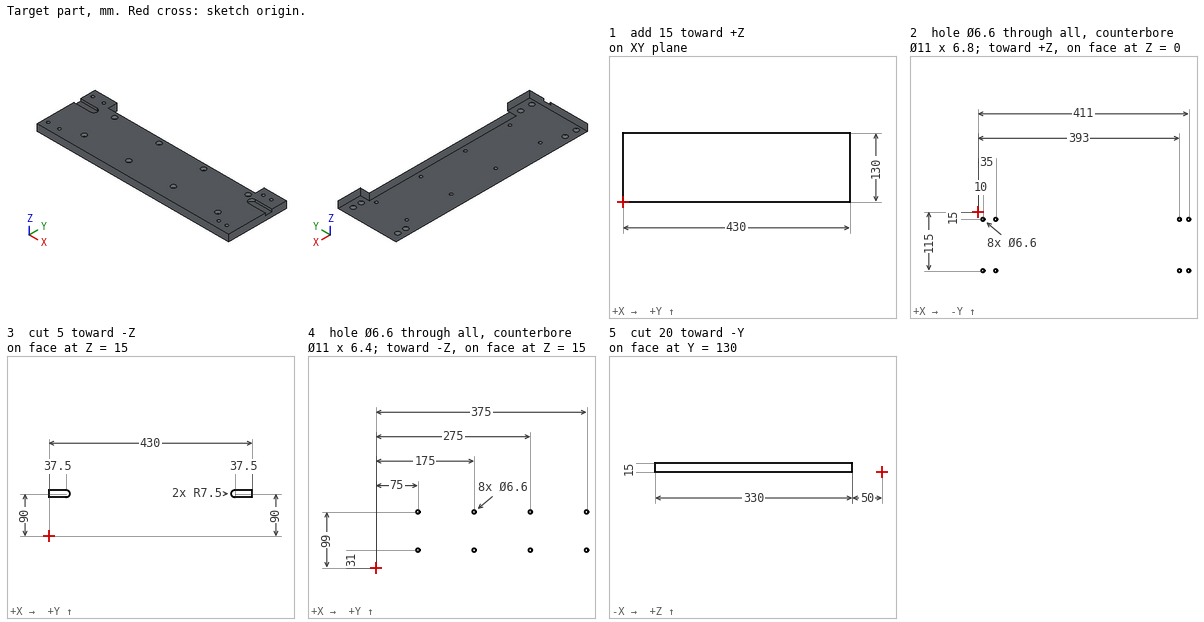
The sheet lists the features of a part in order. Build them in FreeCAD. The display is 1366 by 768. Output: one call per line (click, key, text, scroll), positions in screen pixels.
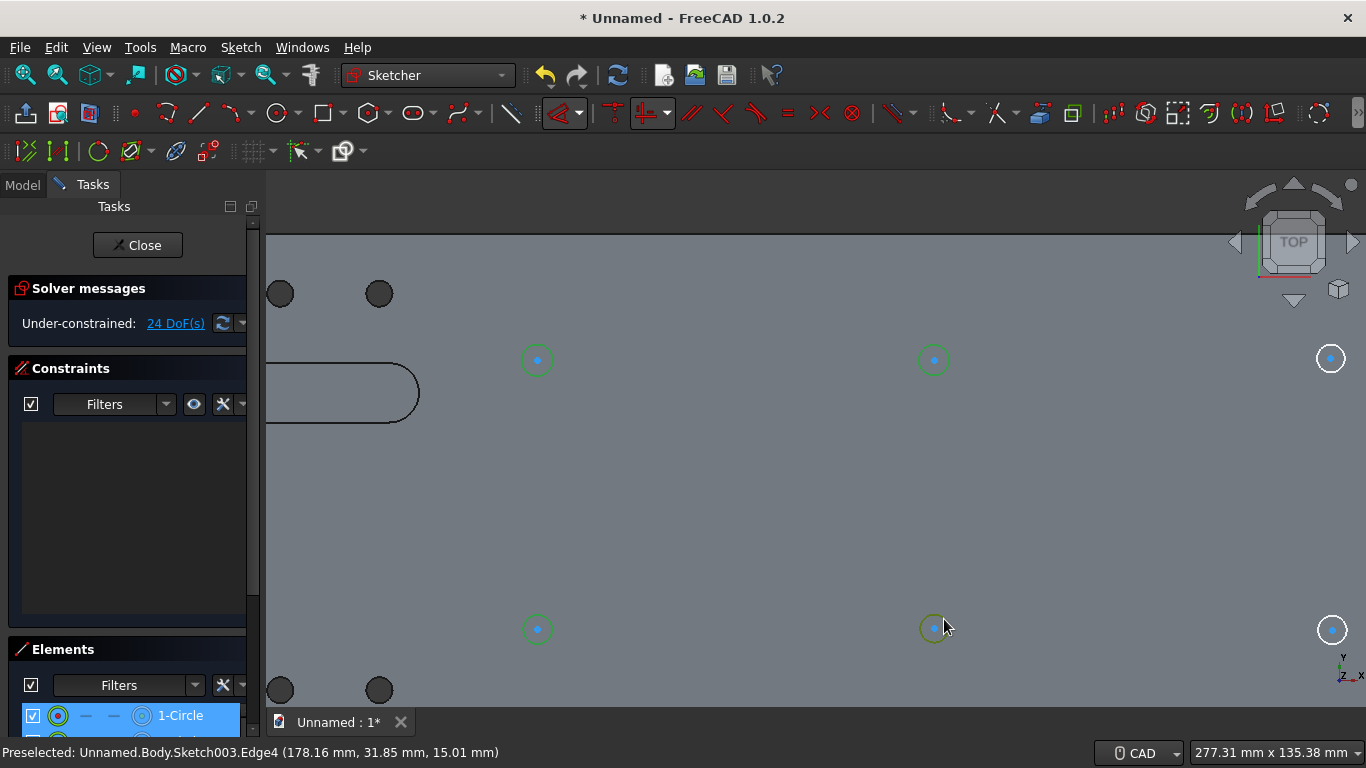
scroll(549, 350, down, 4)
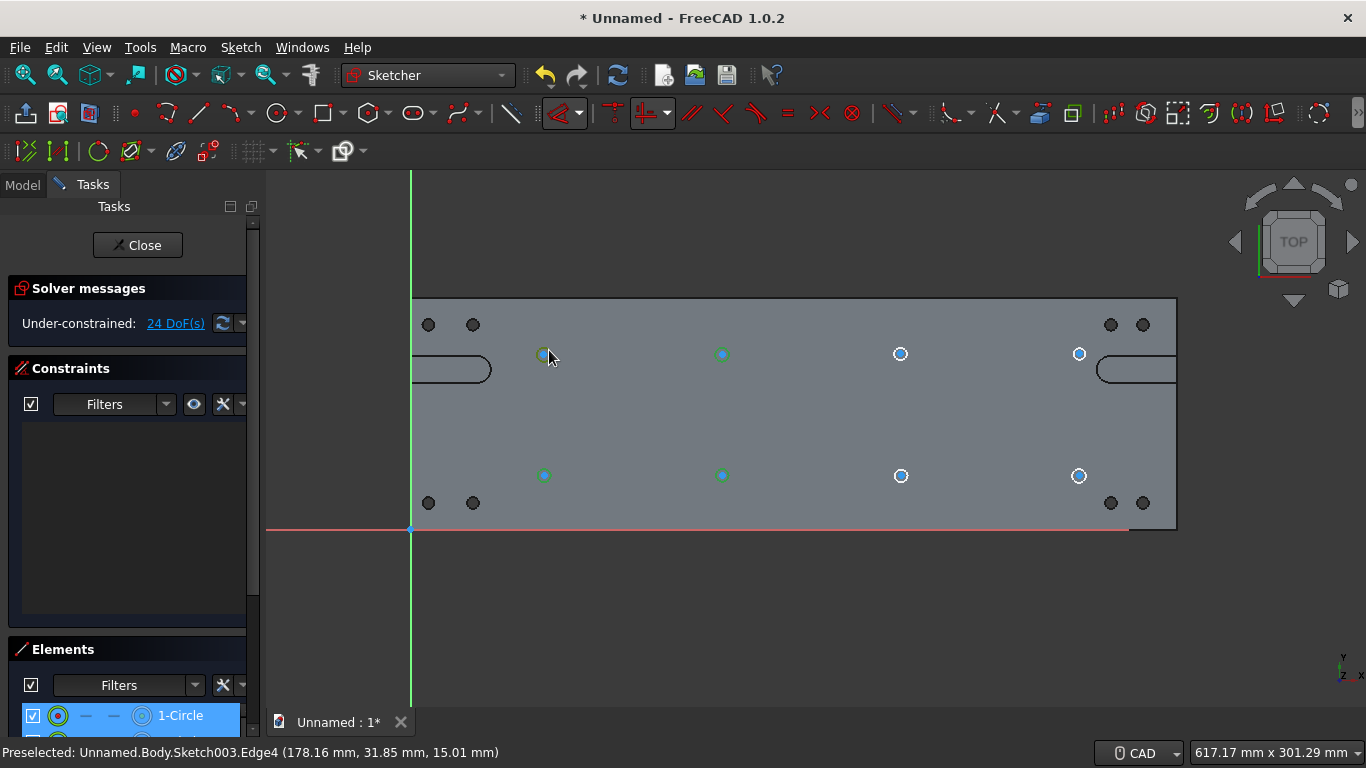
scroll(905, 350, up, 4)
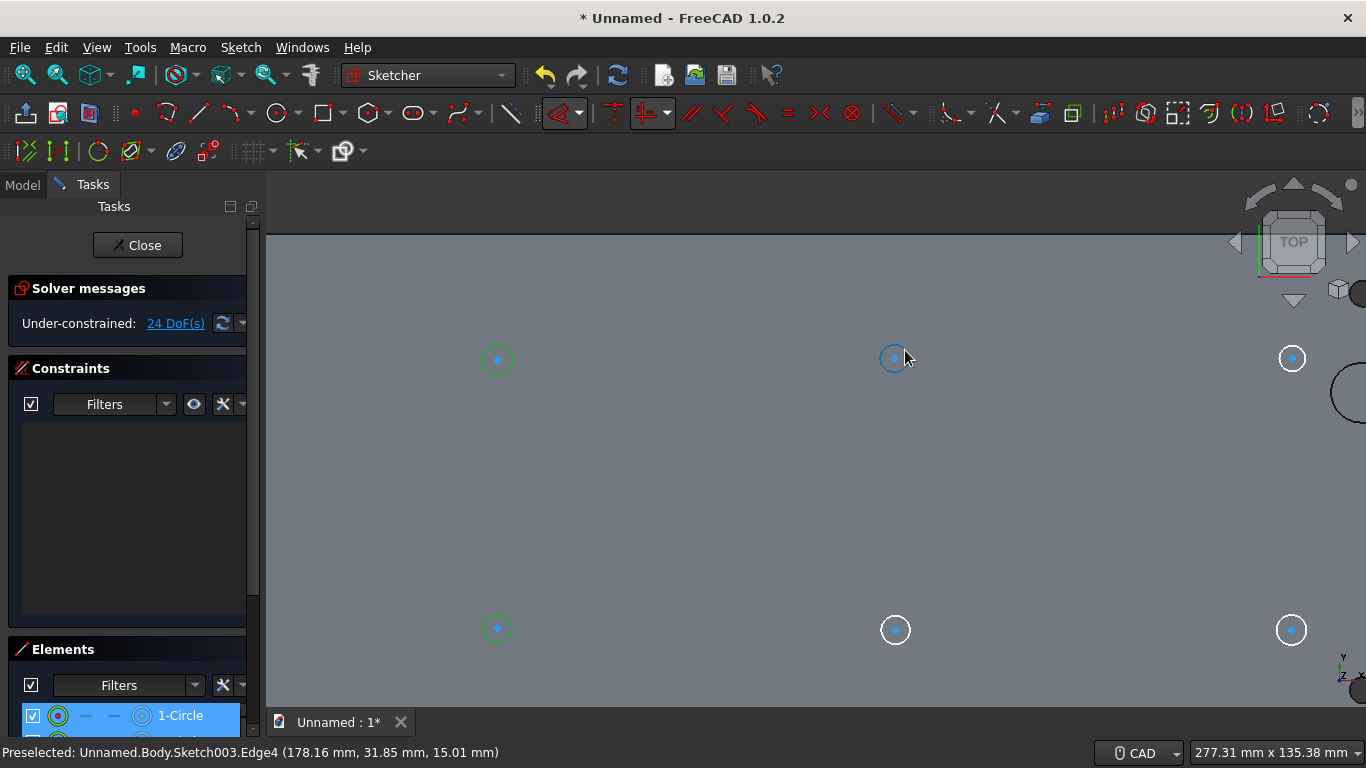
click(904, 349)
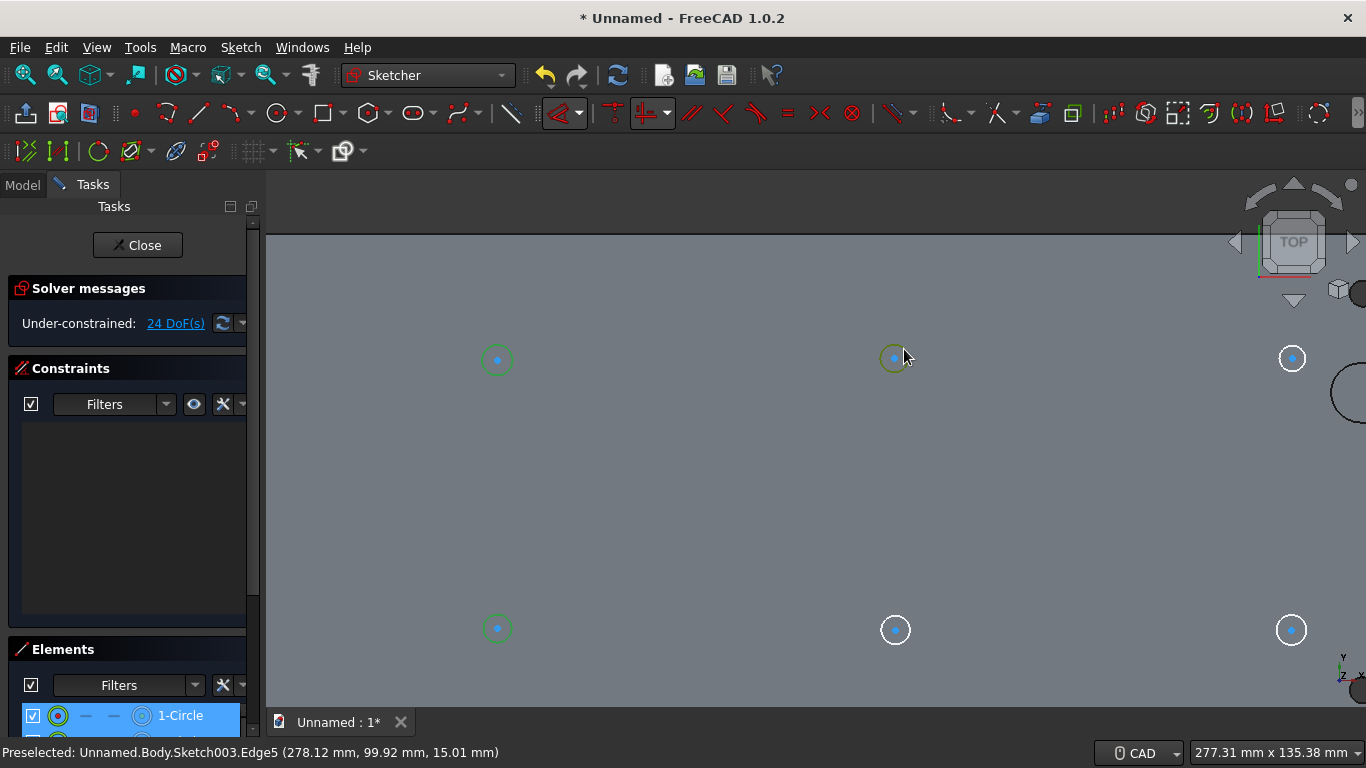
click(906, 620)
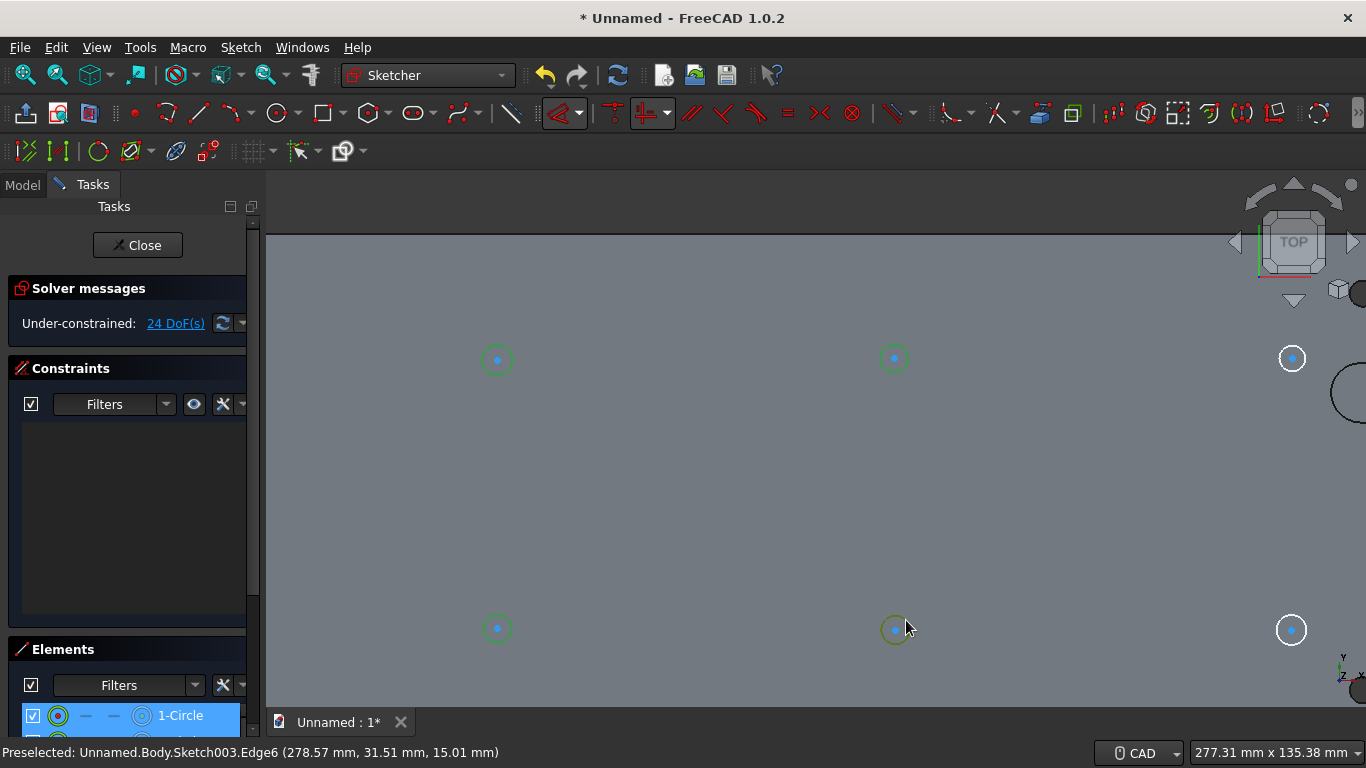
scroll(905, 350, down, 4)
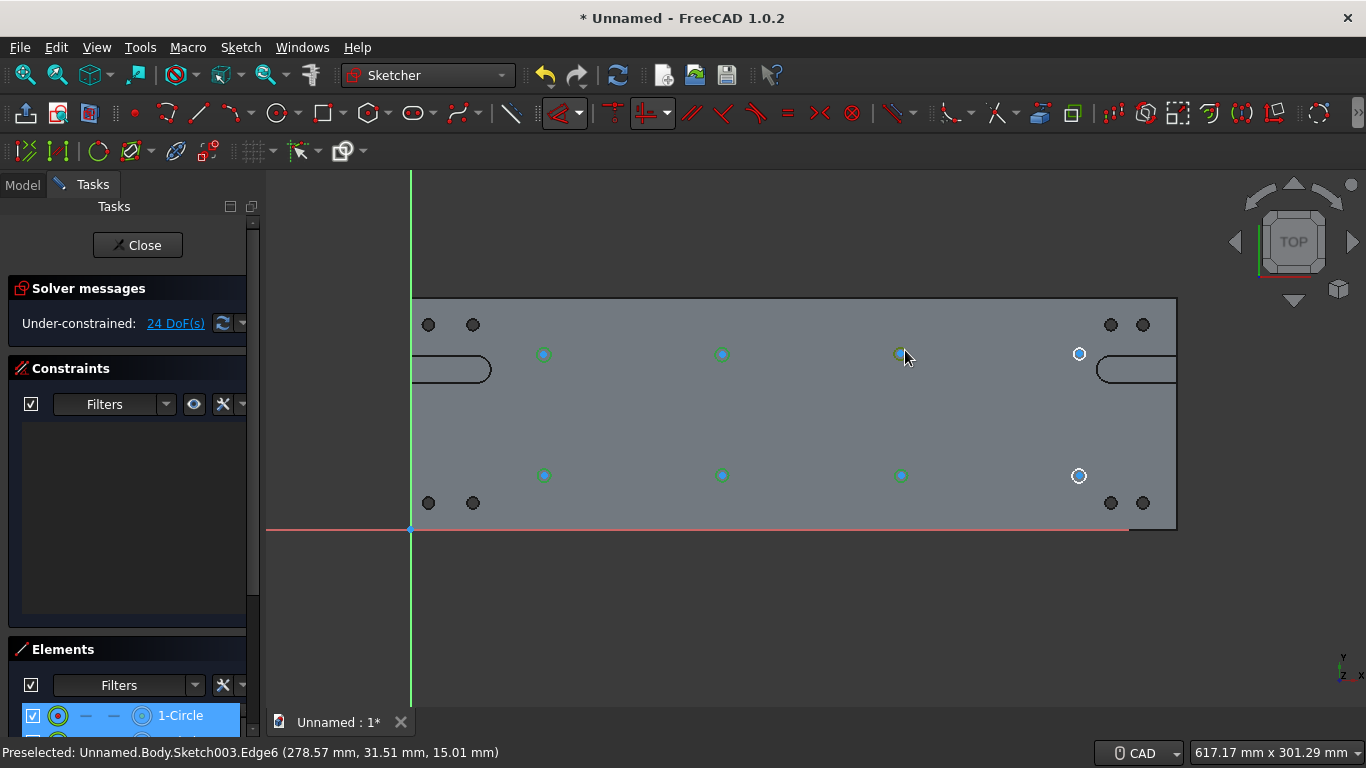
scroll(1083, 350, up, 5)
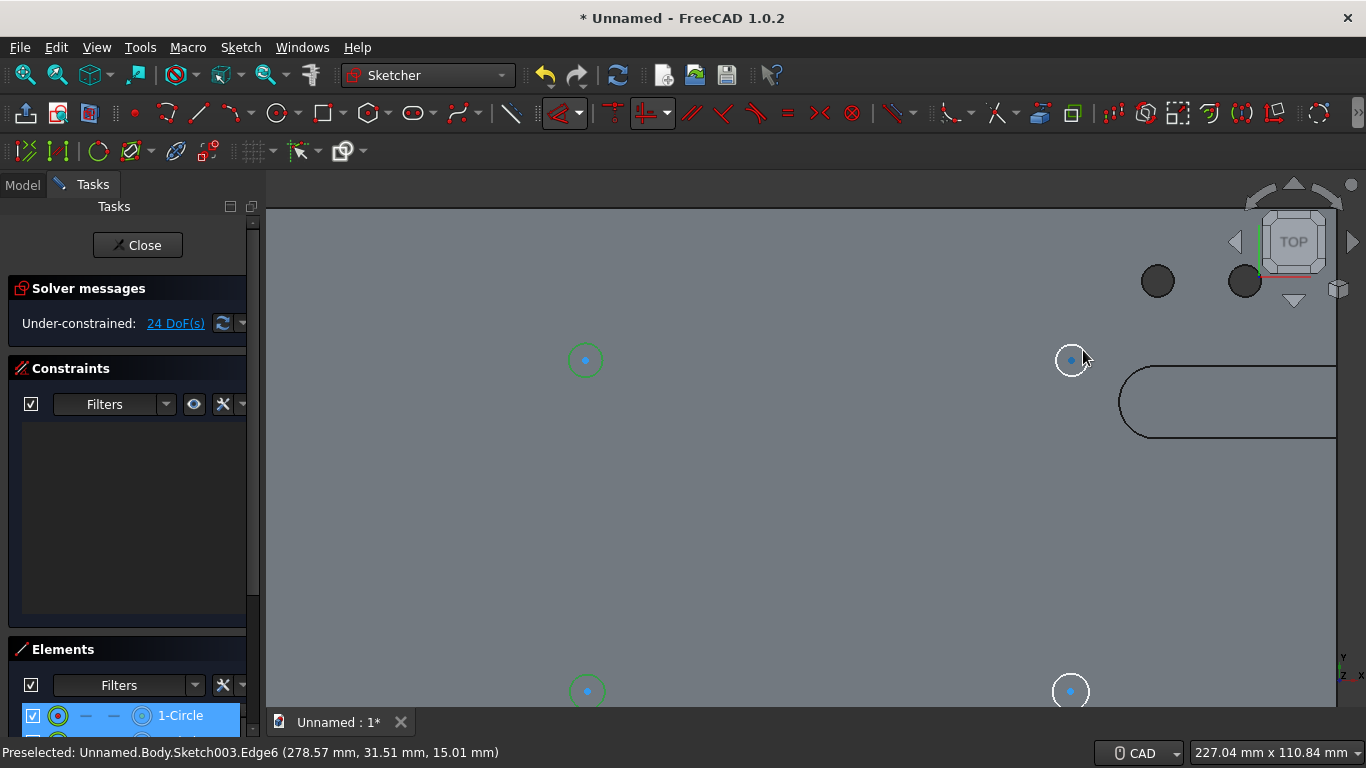
click(1083, 349)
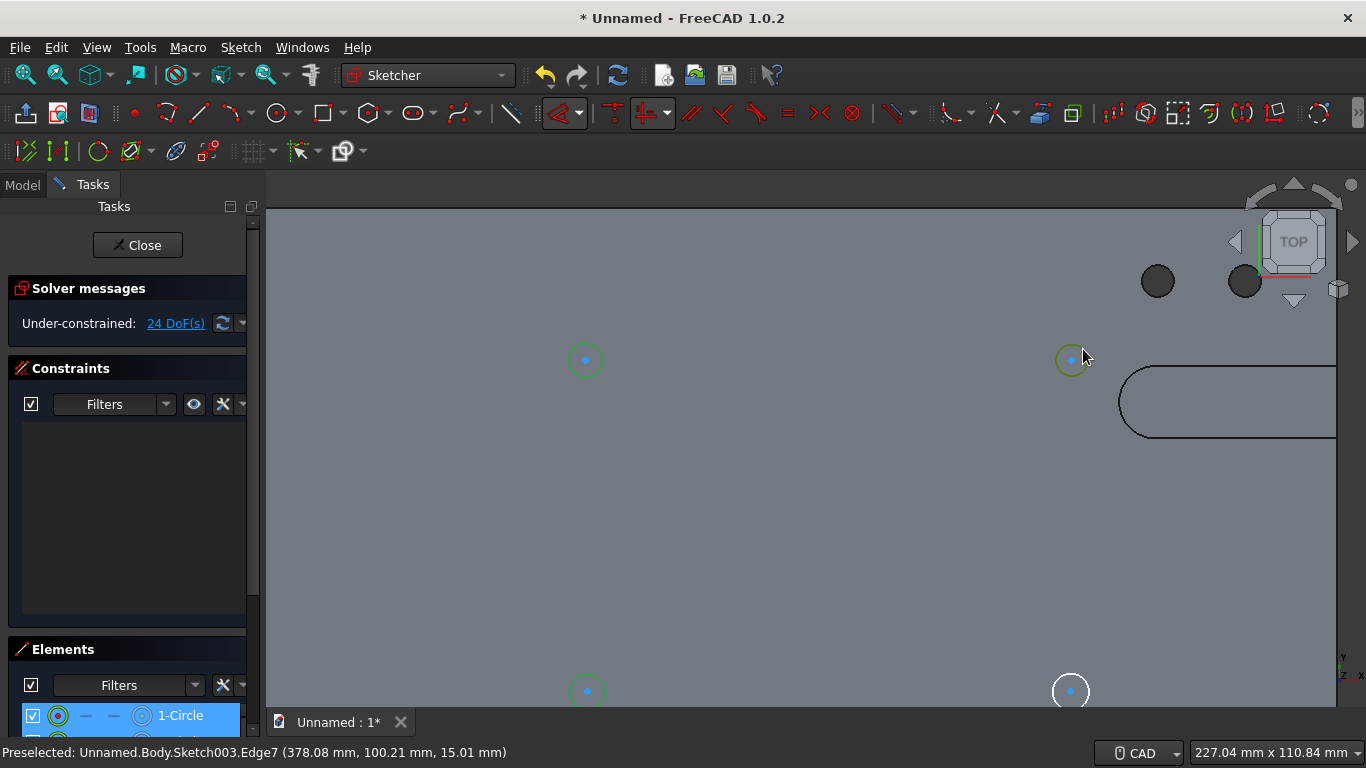
click(1071, 674)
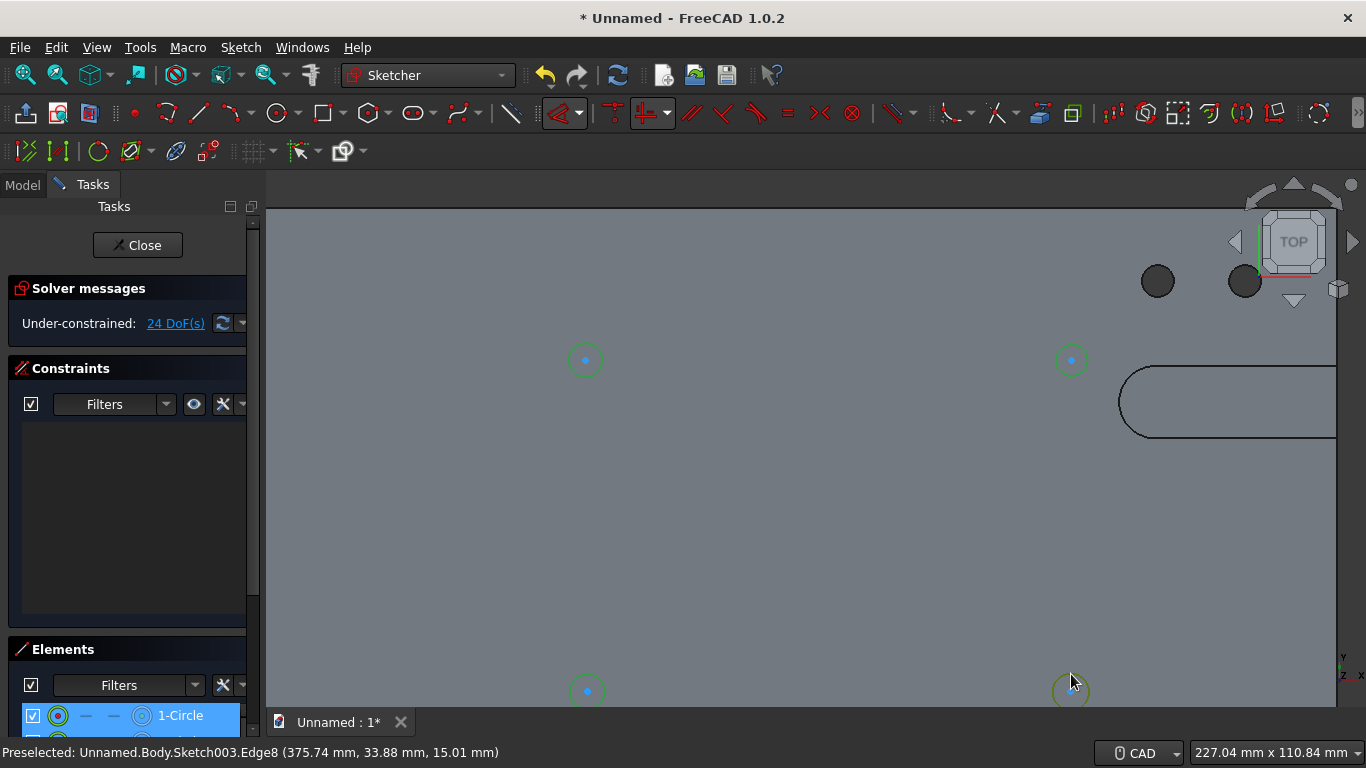
key(e)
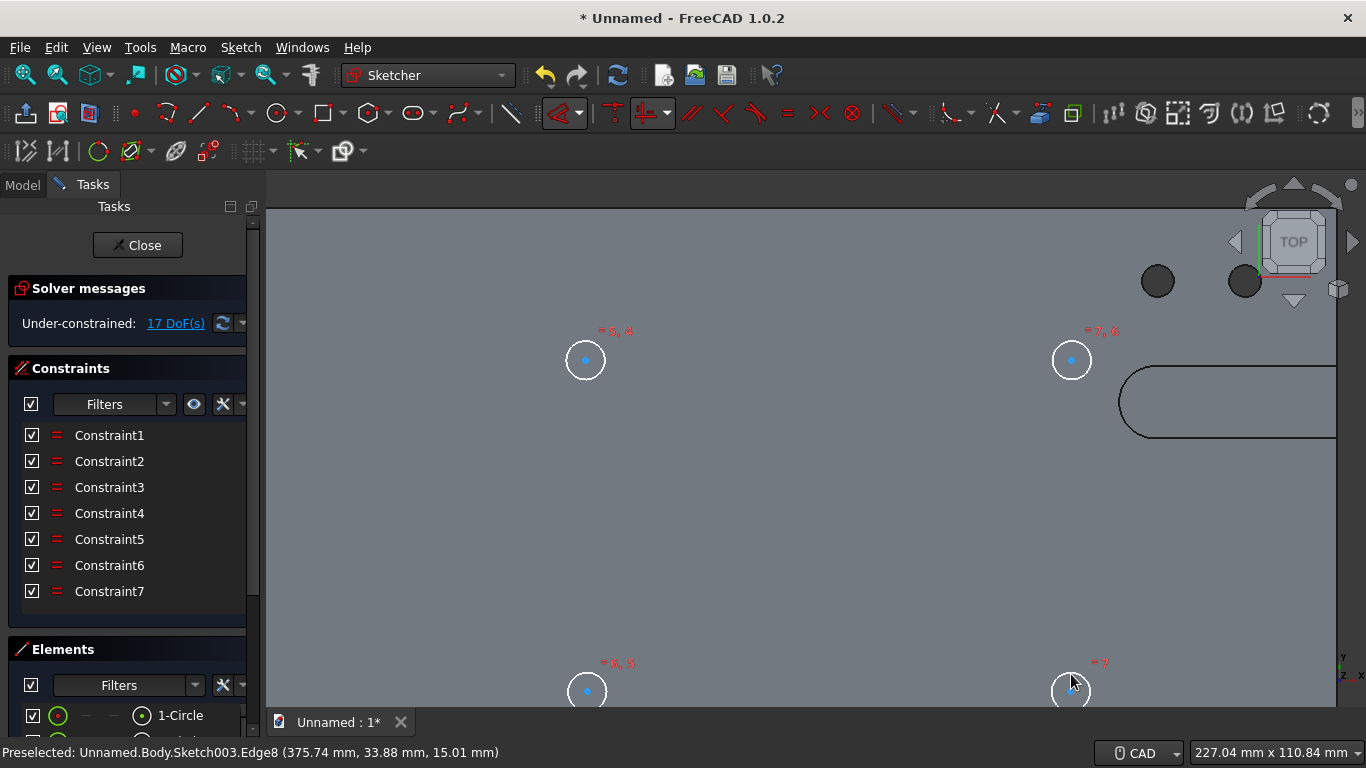
scroll(1083, 350, down, 5)